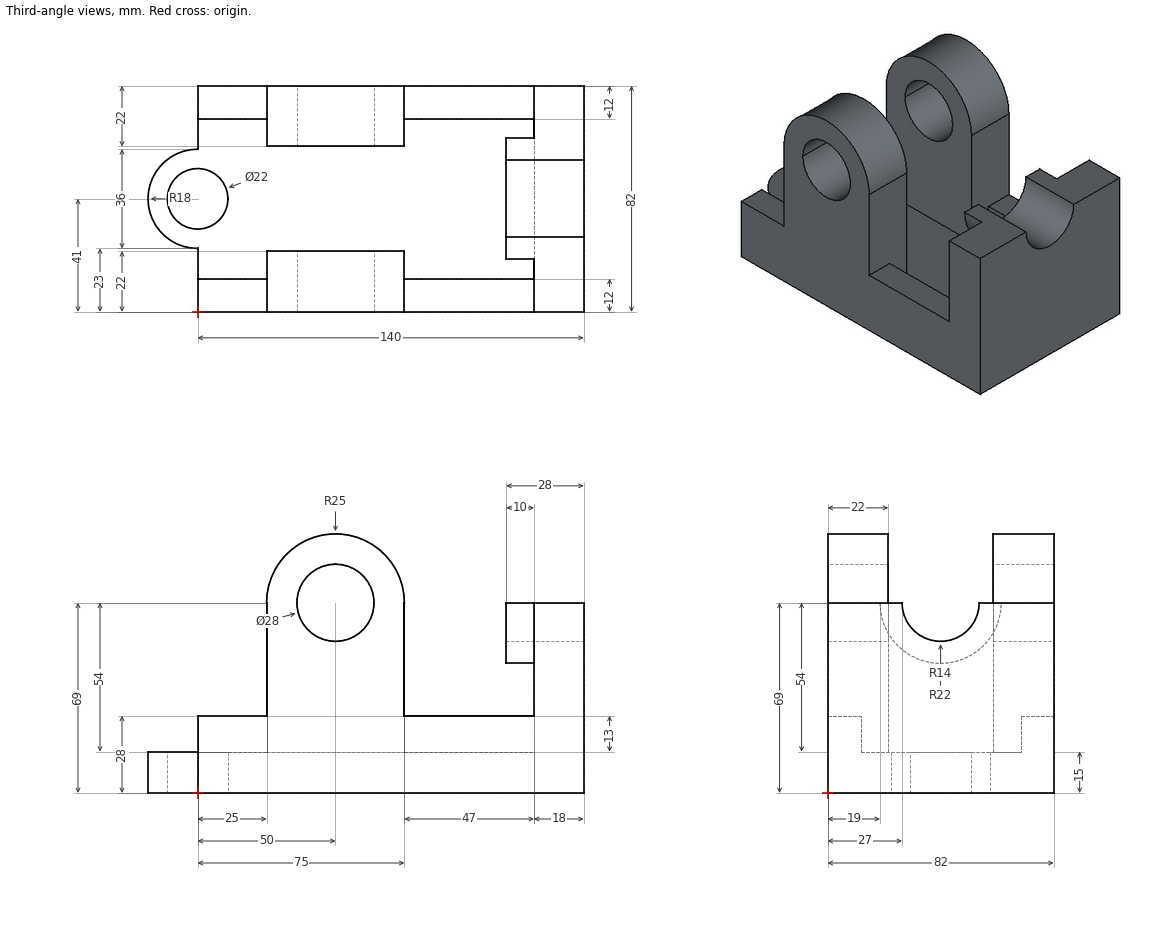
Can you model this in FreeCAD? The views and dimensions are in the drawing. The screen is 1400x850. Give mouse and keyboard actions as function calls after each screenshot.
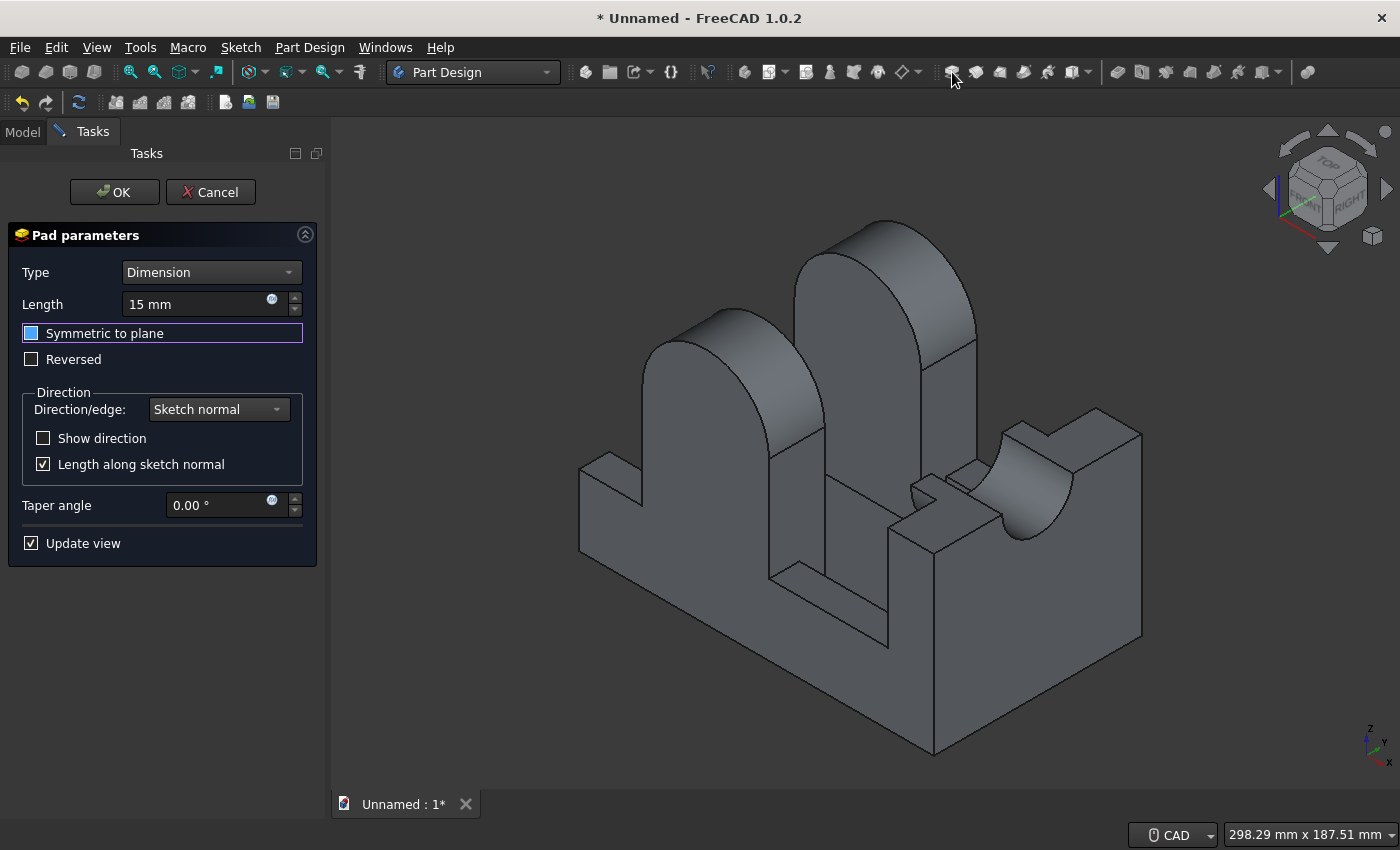
click(30, 359)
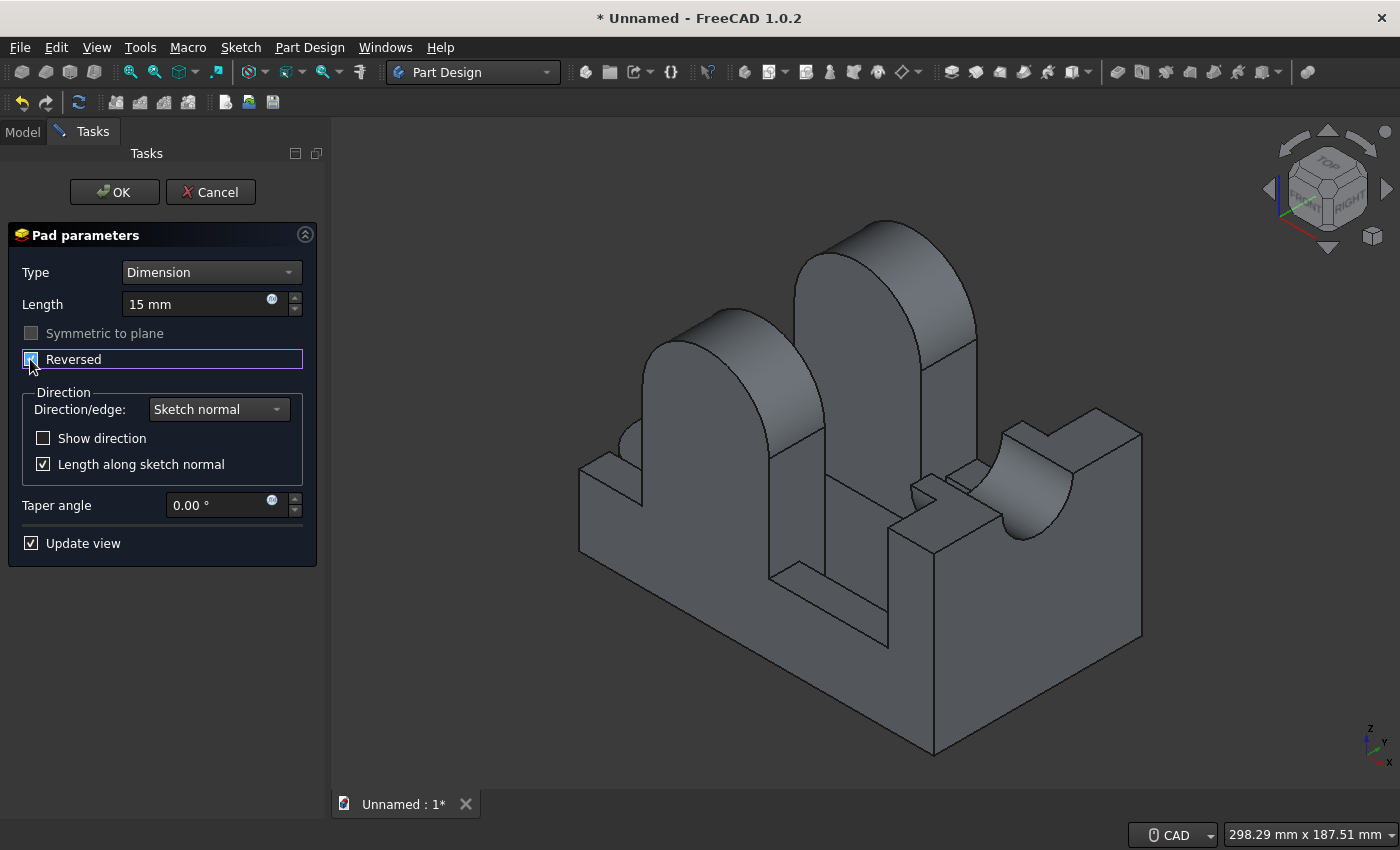
click(115, 192)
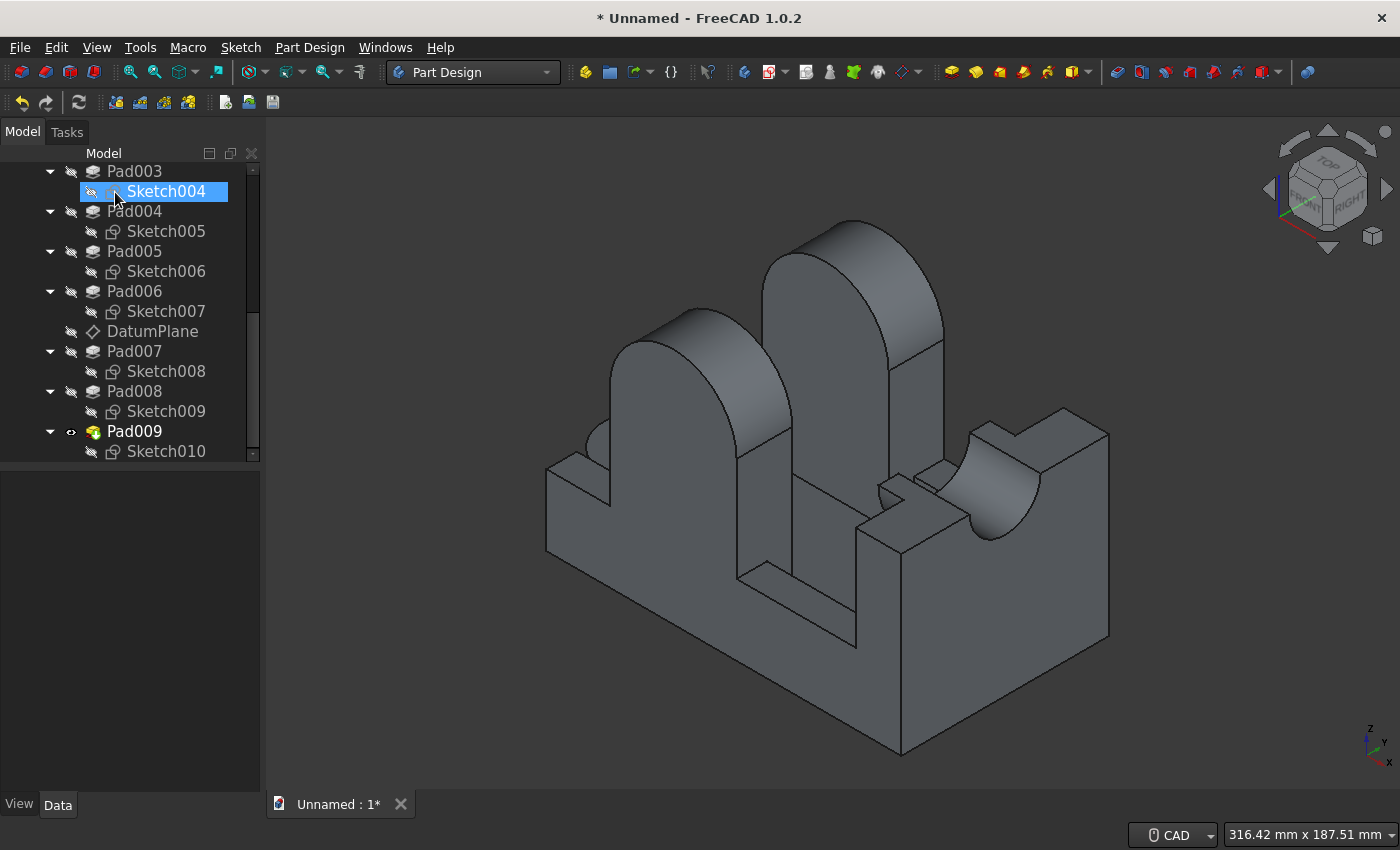
click(833, 552)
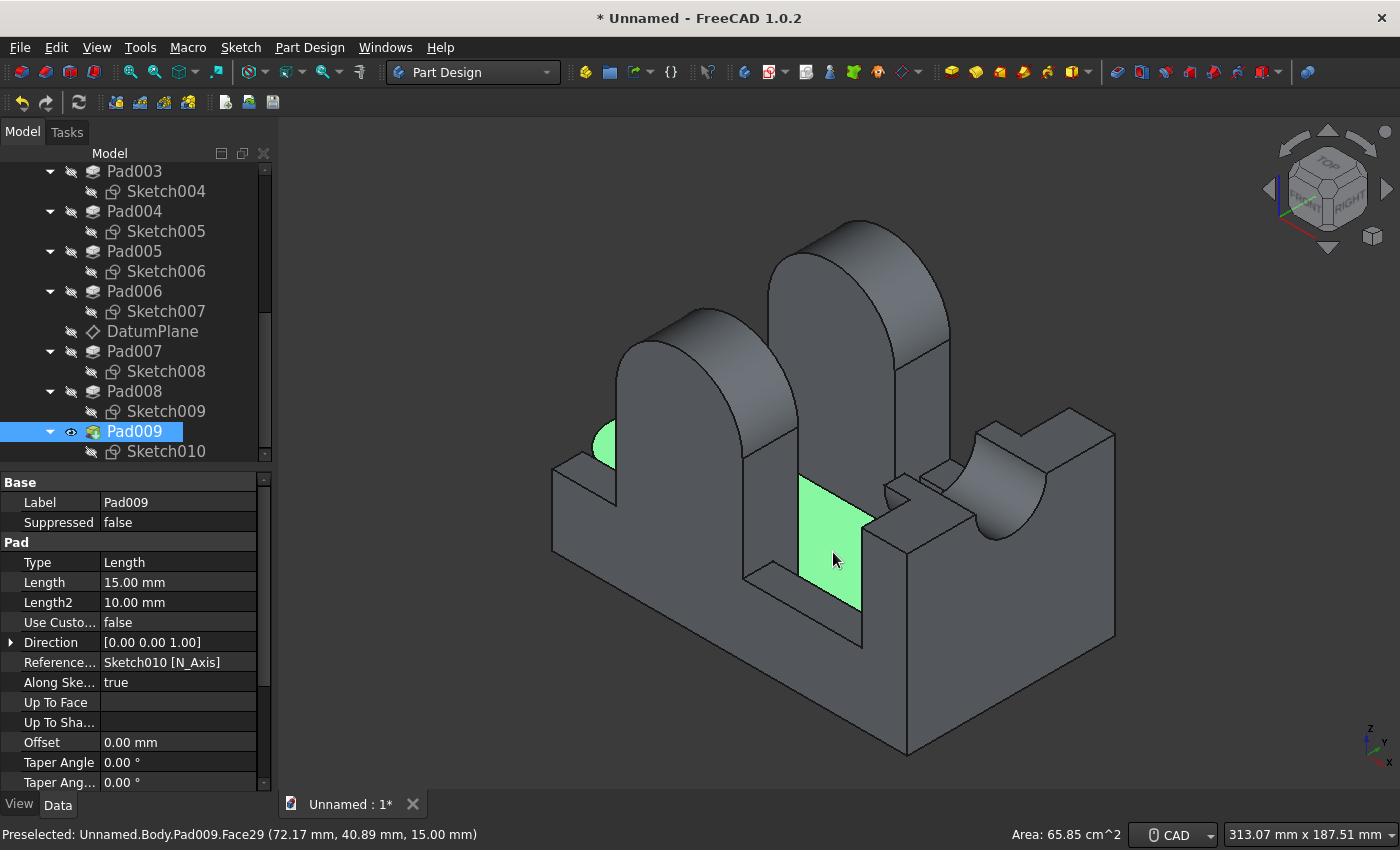
click(770, 72)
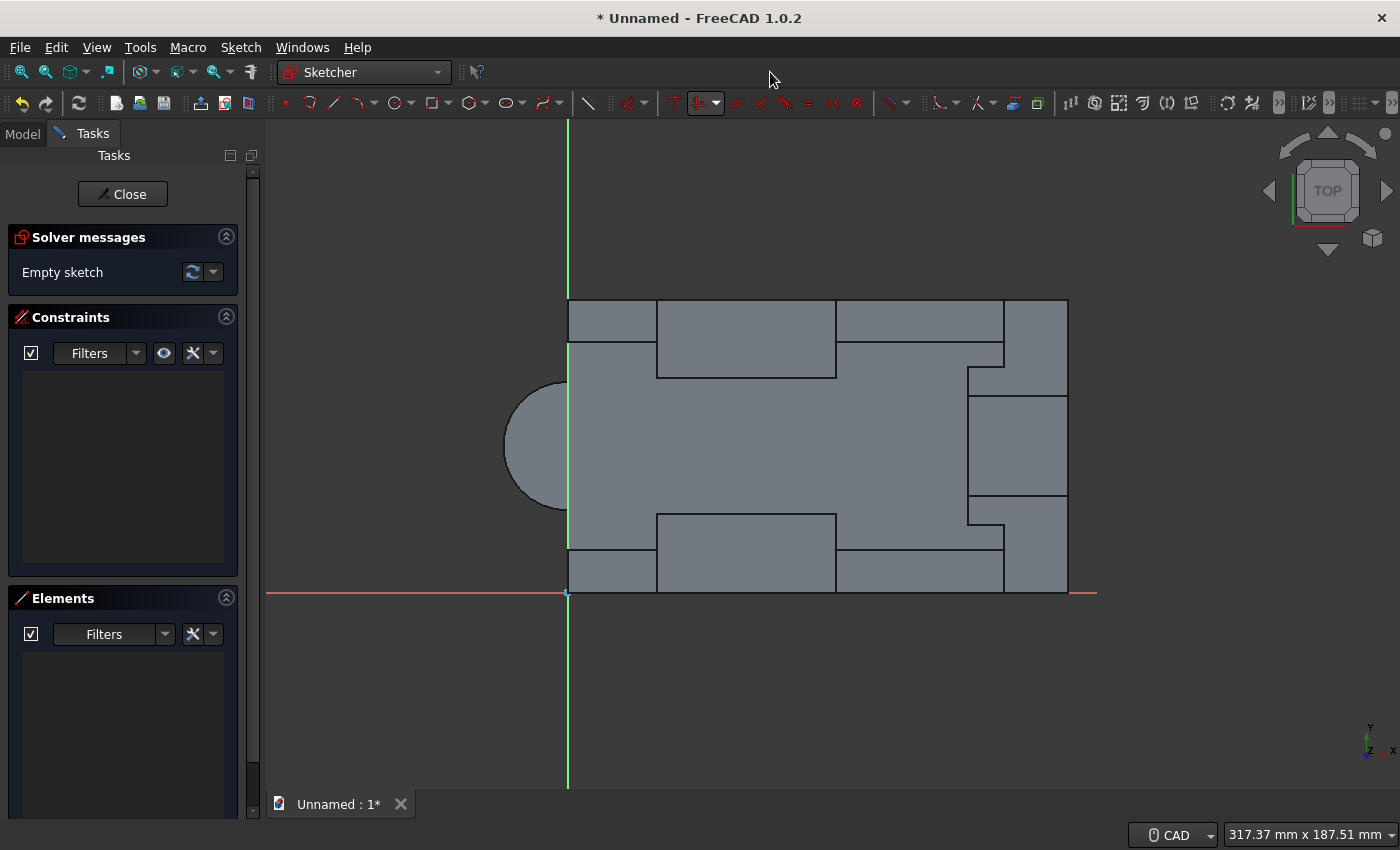
click(250, 104)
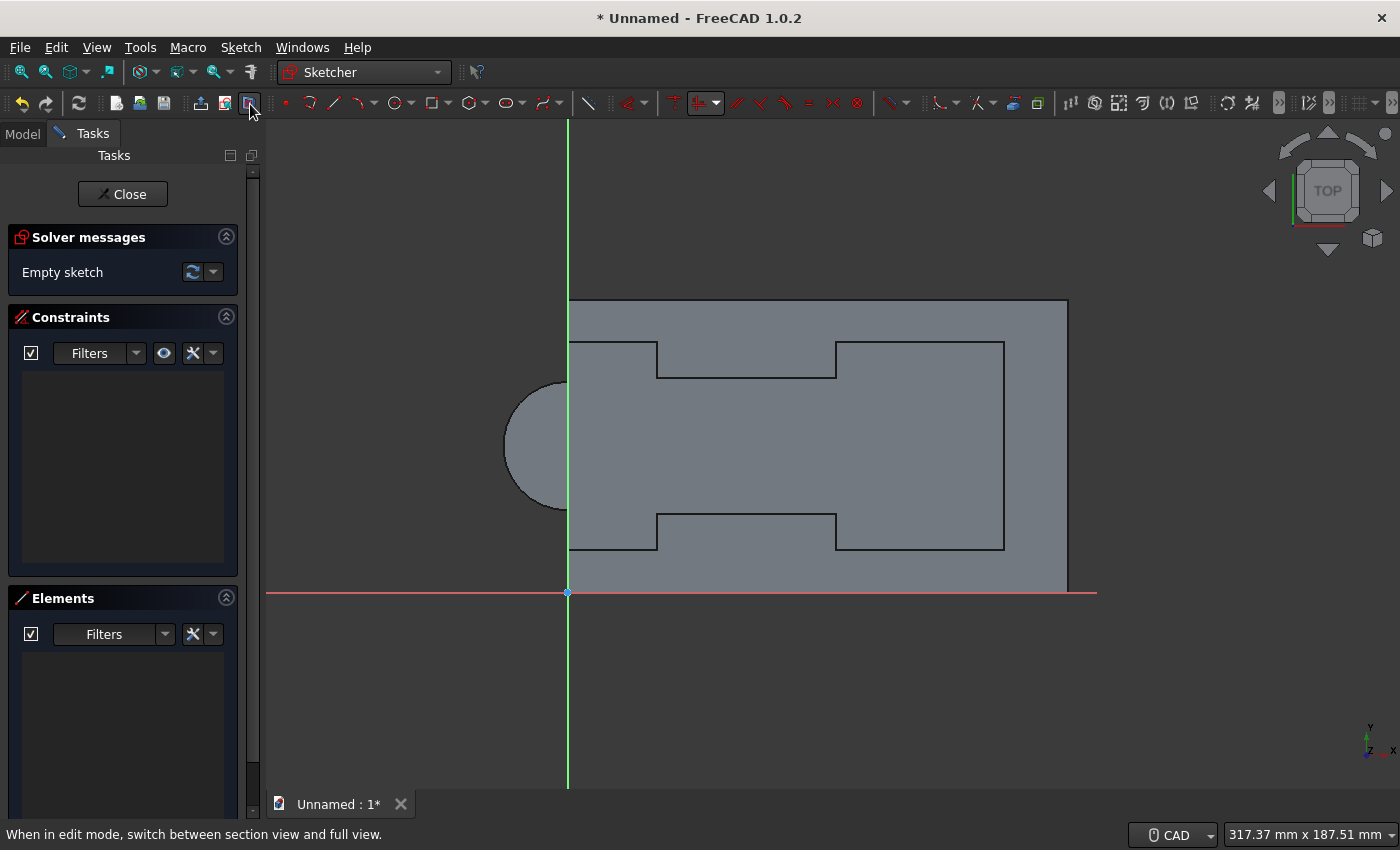
scroll(407, 537, up, 4)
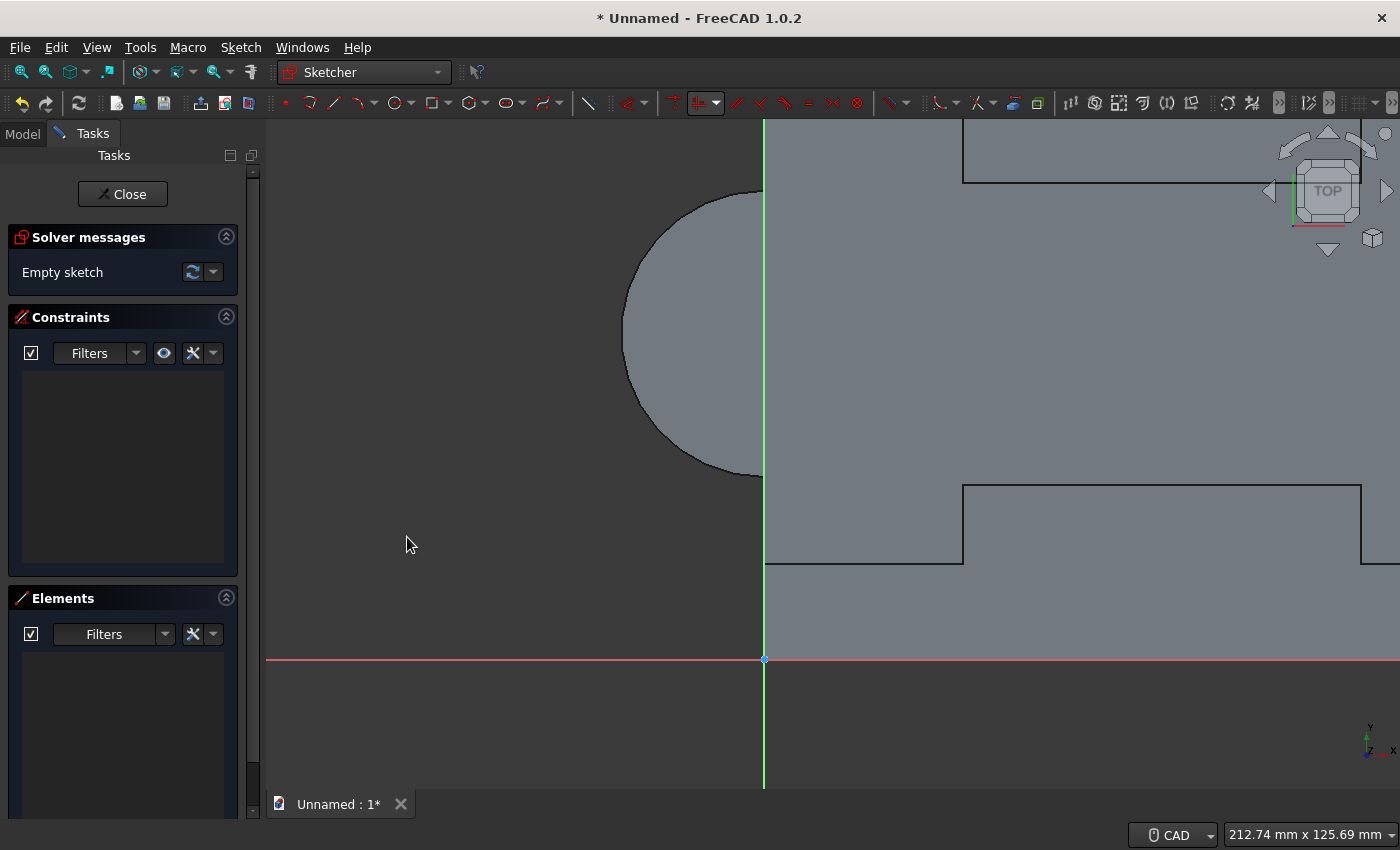
click(396, 104)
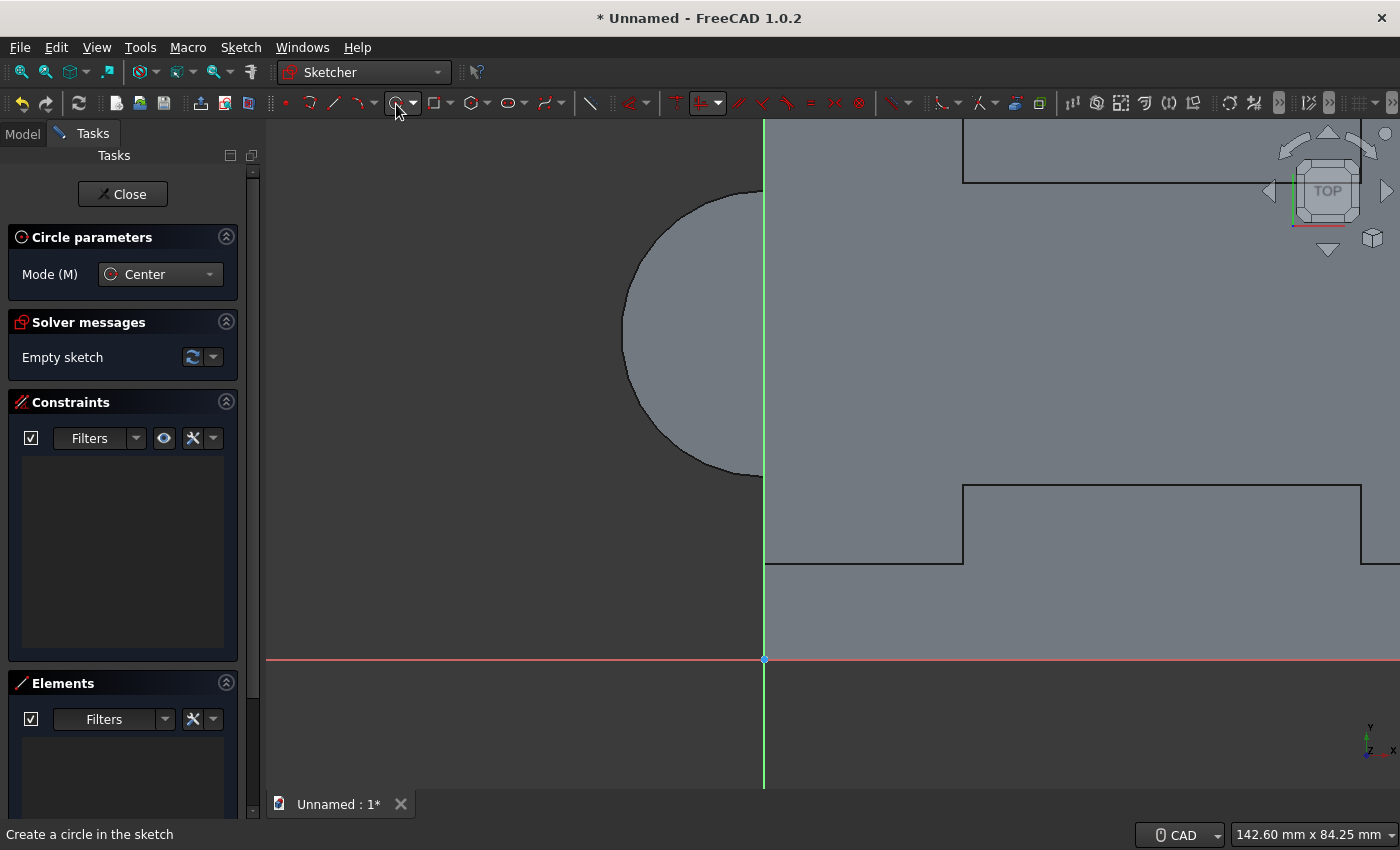
click(764, 334)
click(826, 272)
key(Escape)